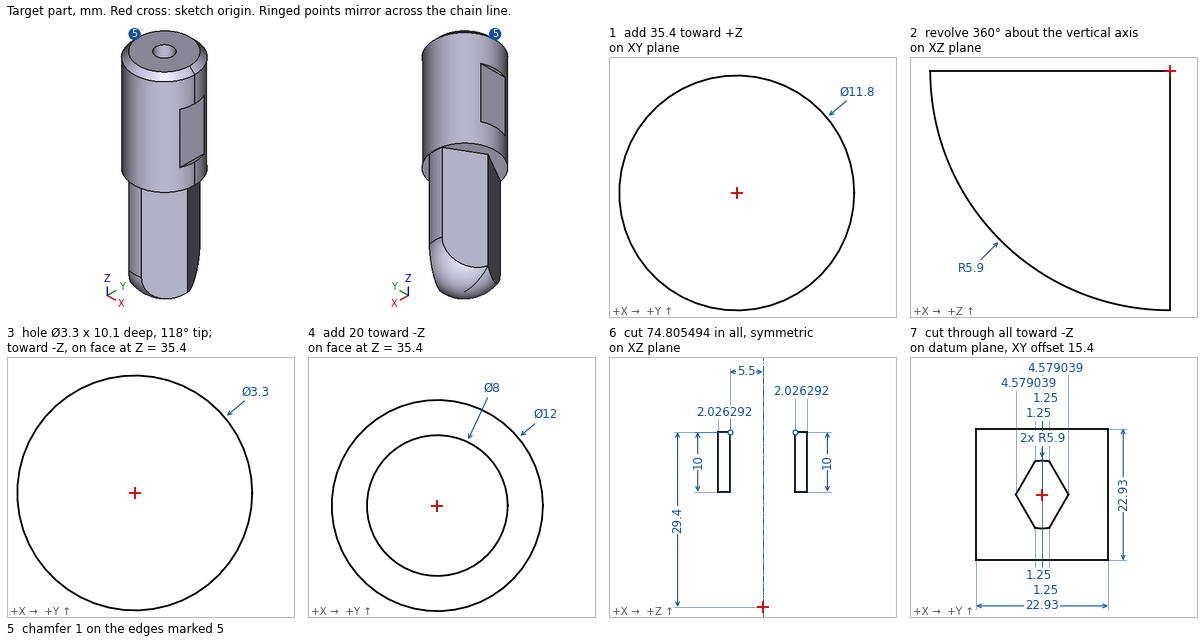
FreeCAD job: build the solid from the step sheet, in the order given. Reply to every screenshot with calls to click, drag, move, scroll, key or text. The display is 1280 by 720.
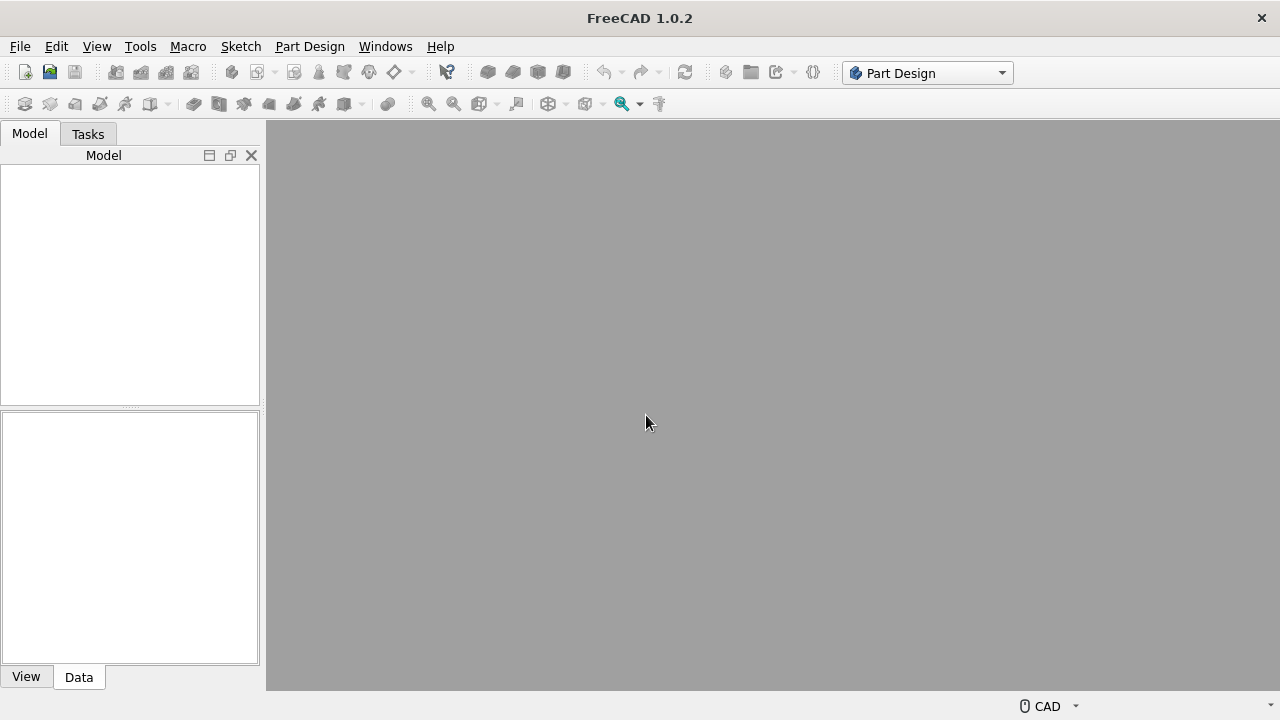
click(25, 72)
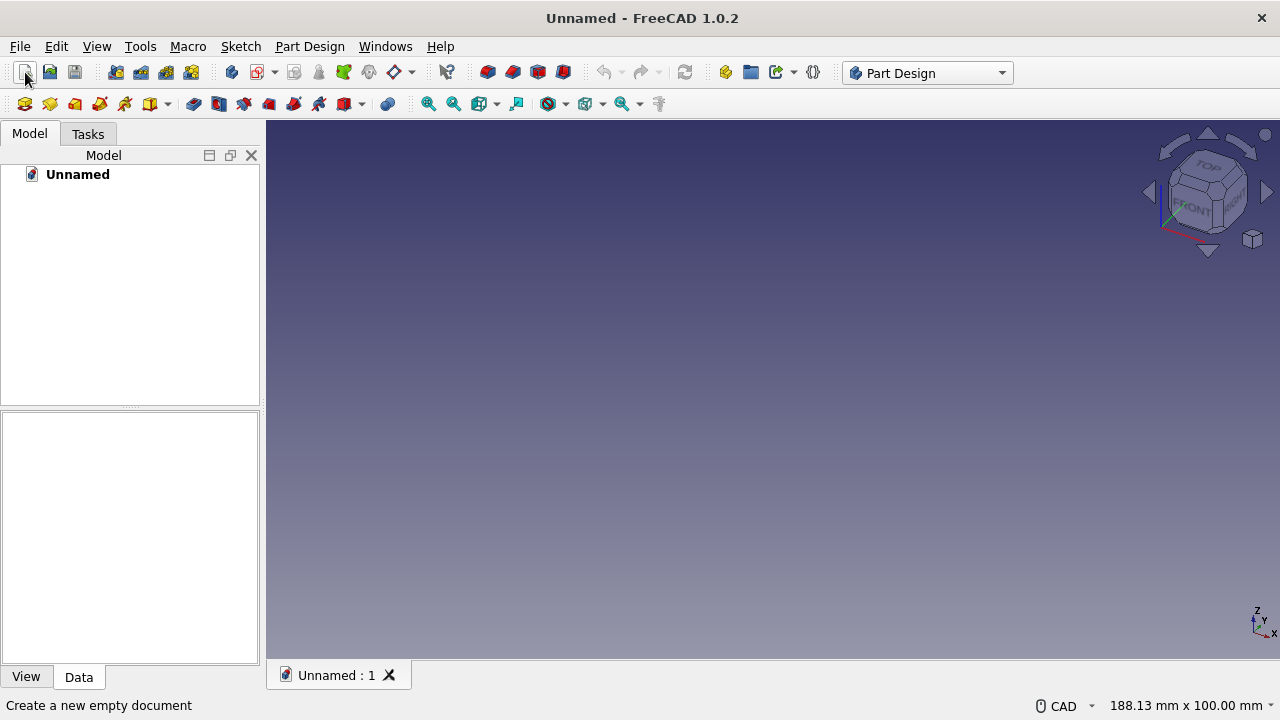
click(256, 72)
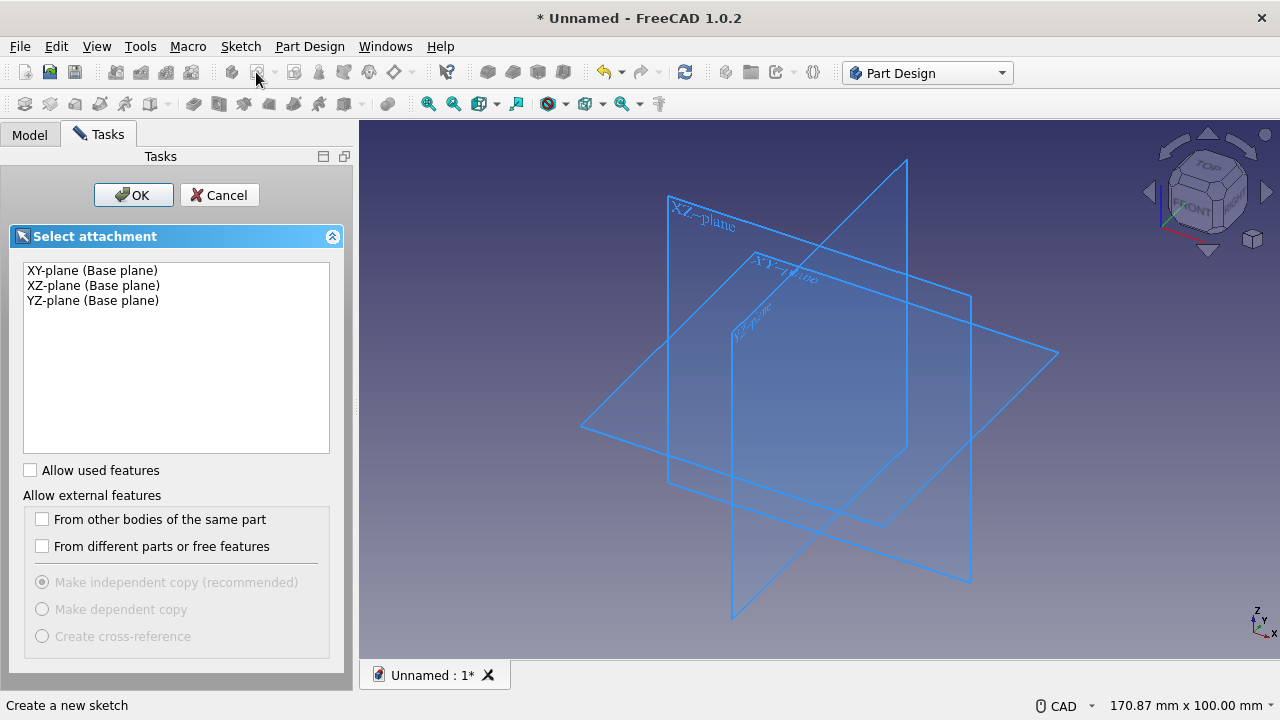
click(84, 270)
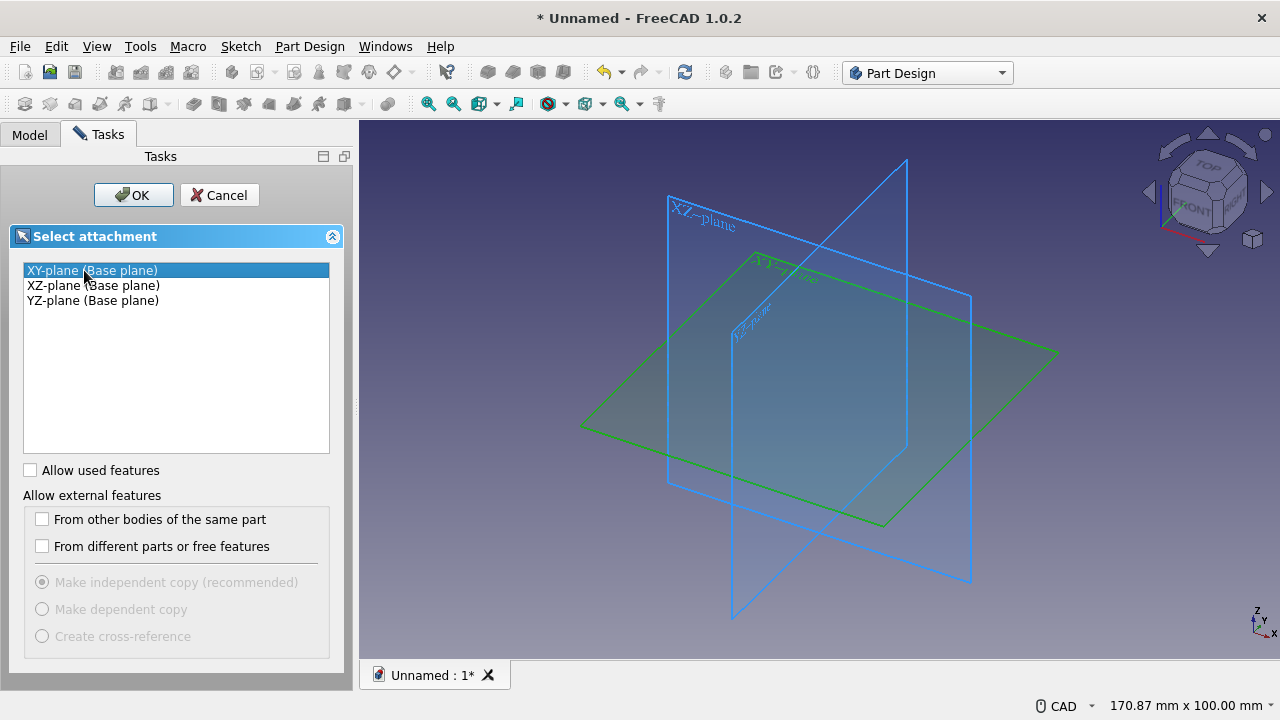
click(134, 195)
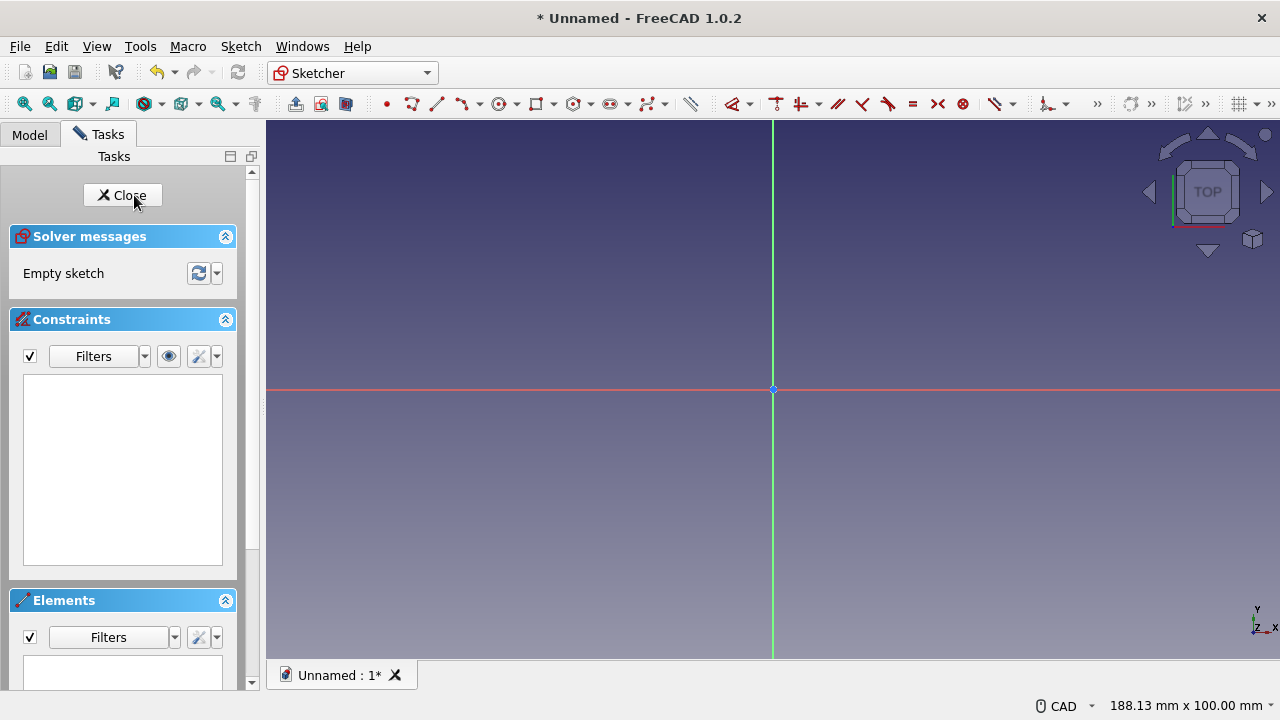
scroll(790, 390, up, 8)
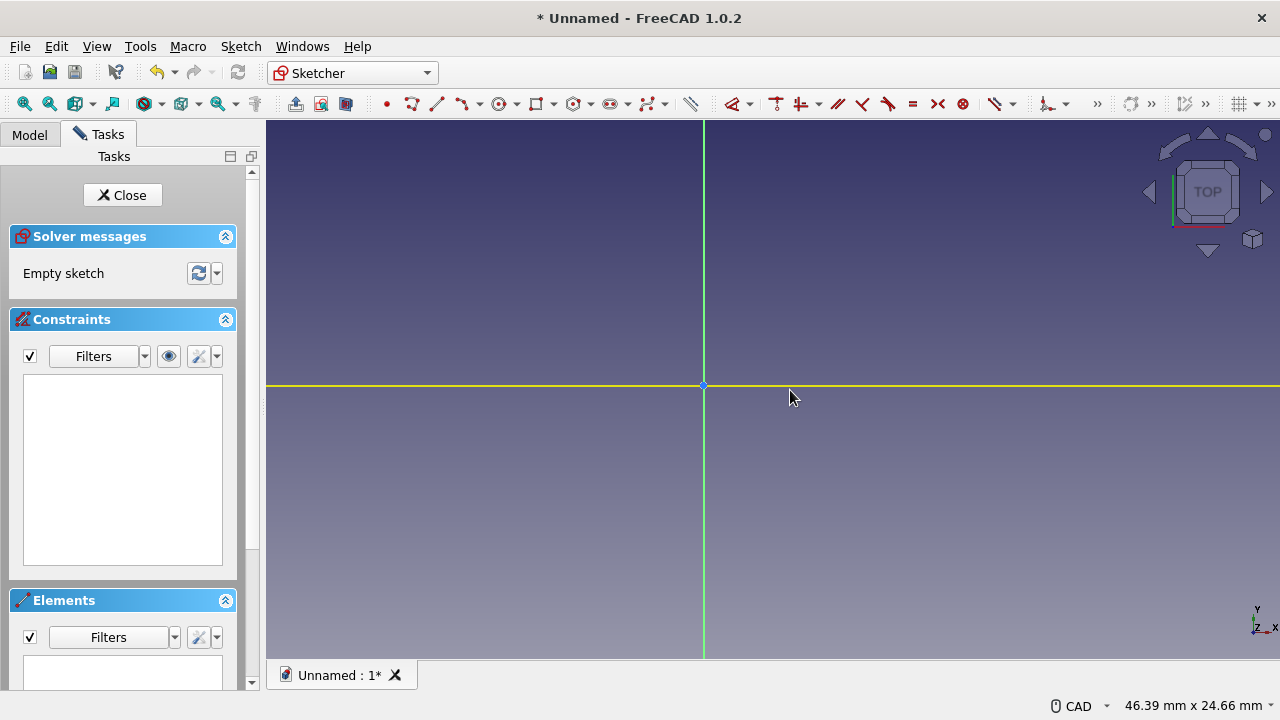
key(g)
key(c)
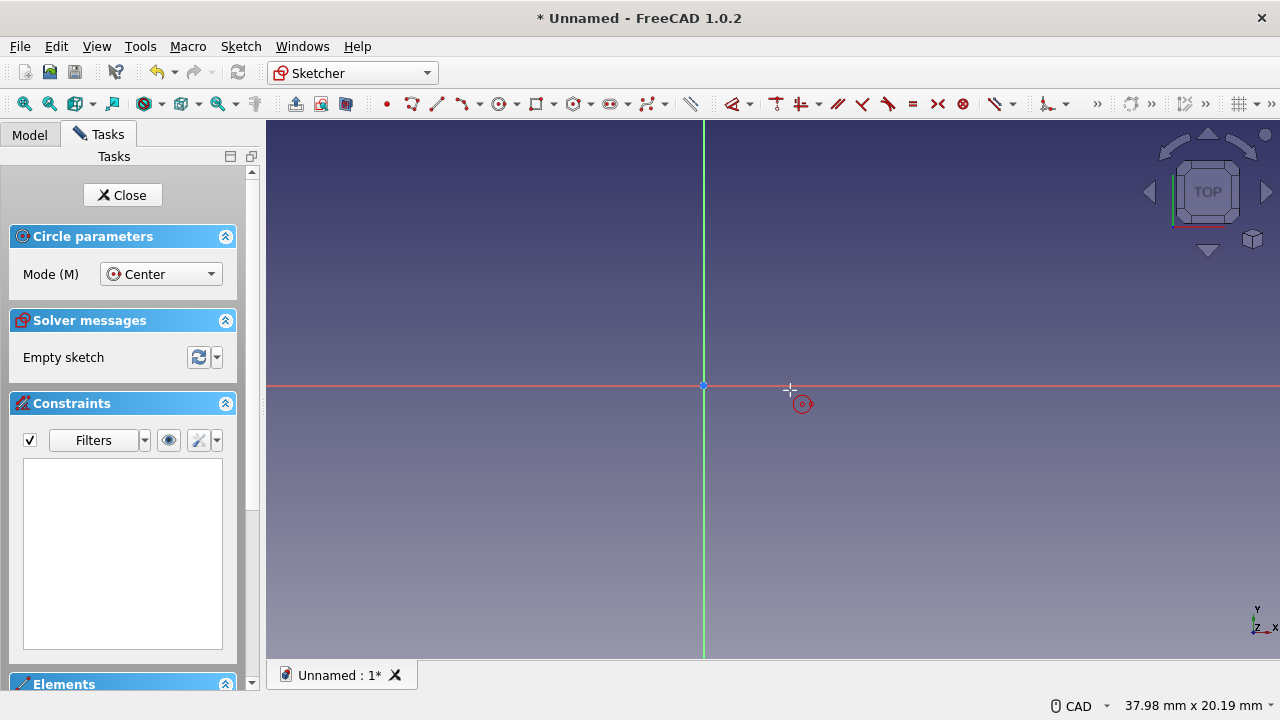
click(704, 386)
move(815, 274)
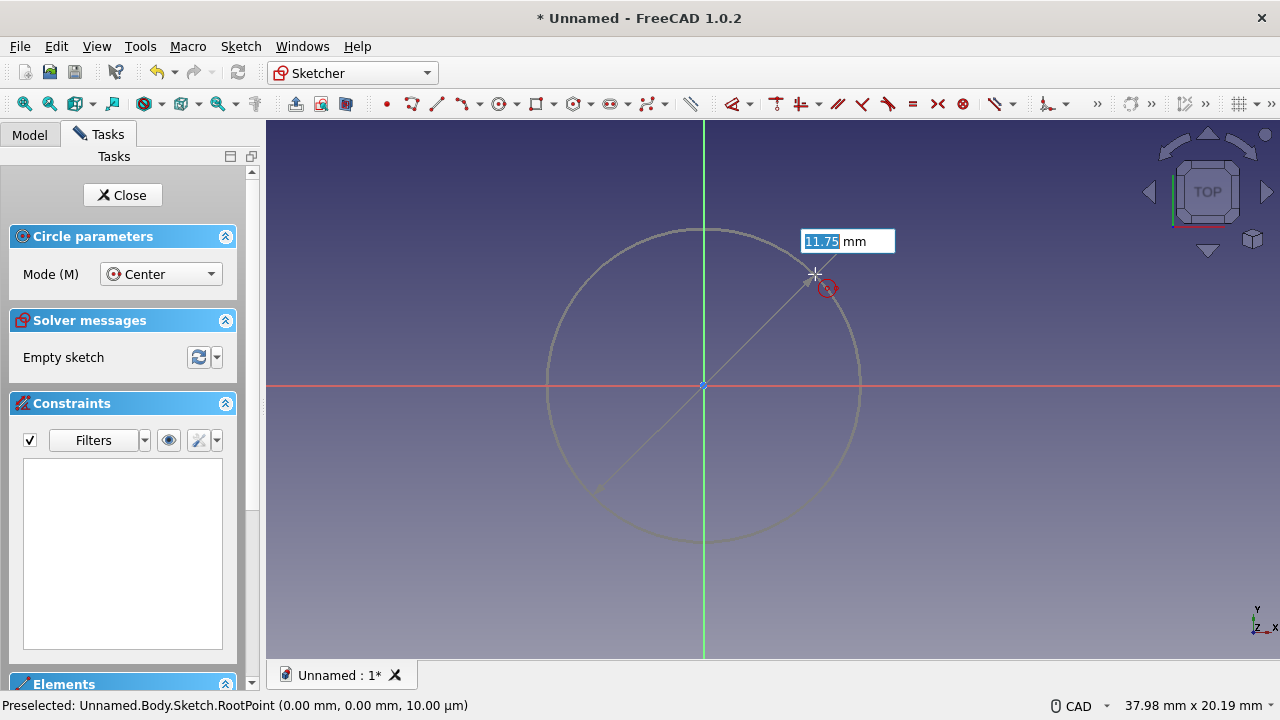
text(11.8)
key(Return)
key(Escape)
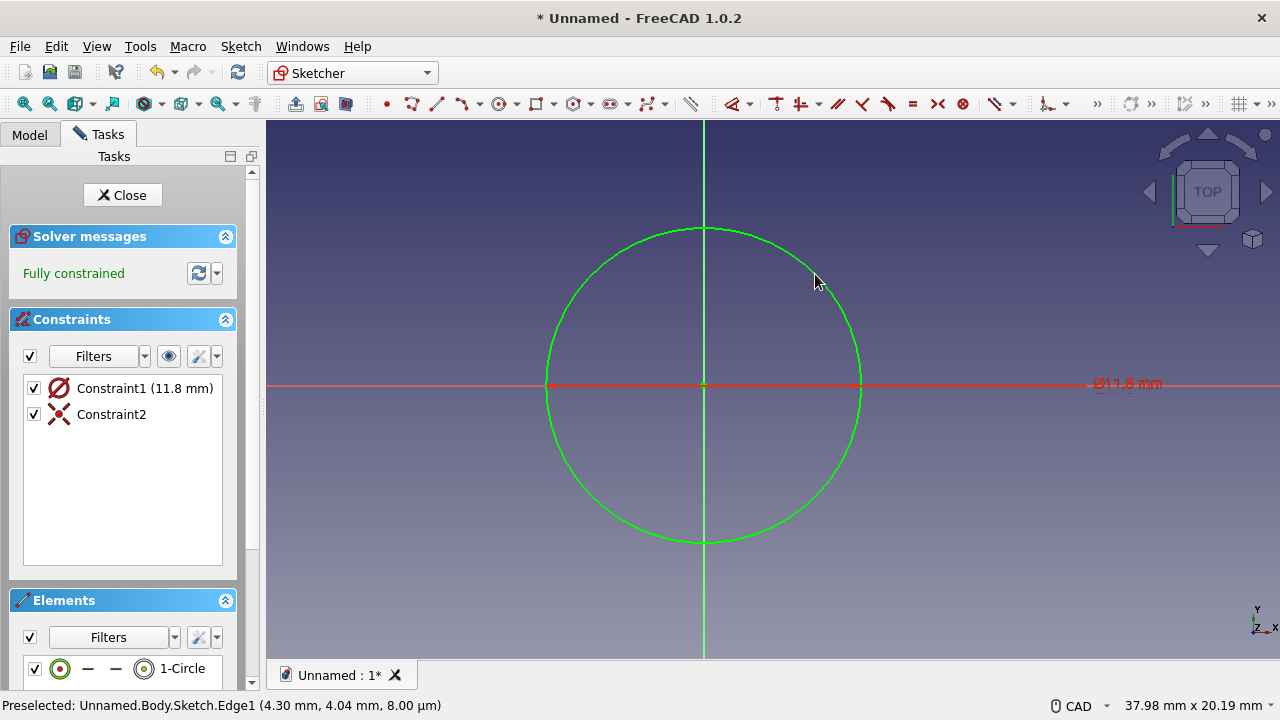
click(123, 195)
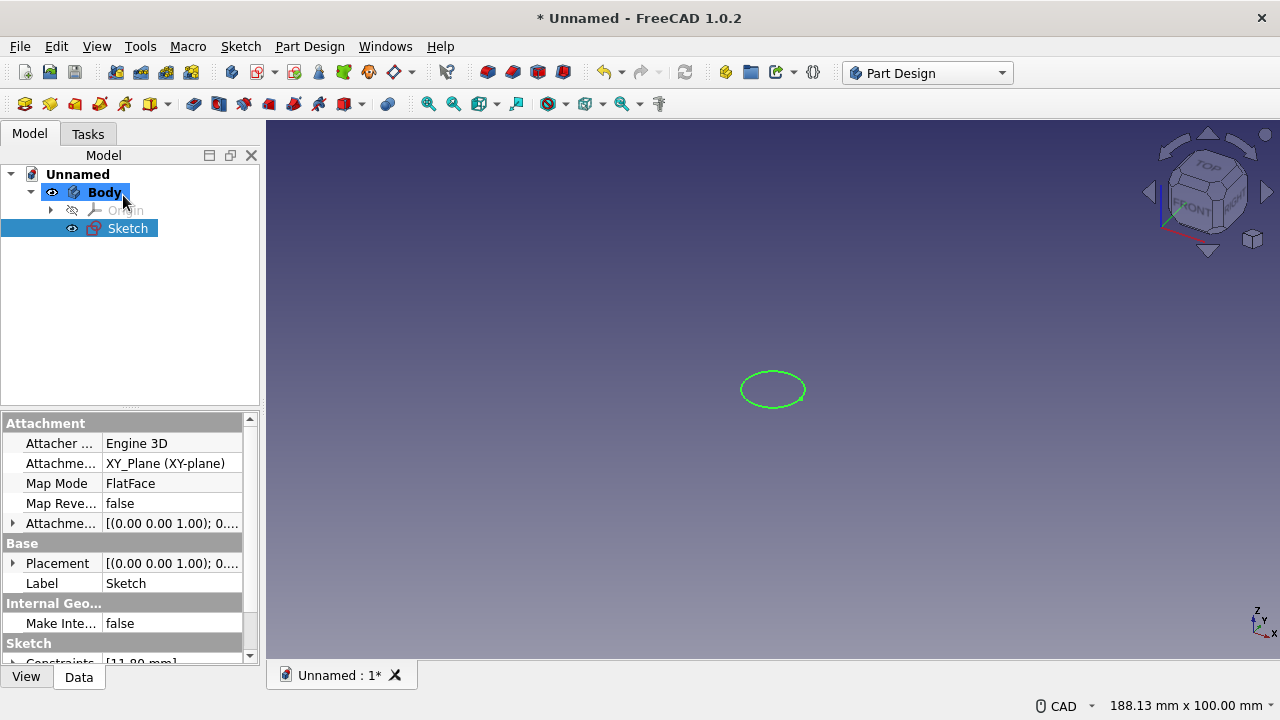
click(25, 104)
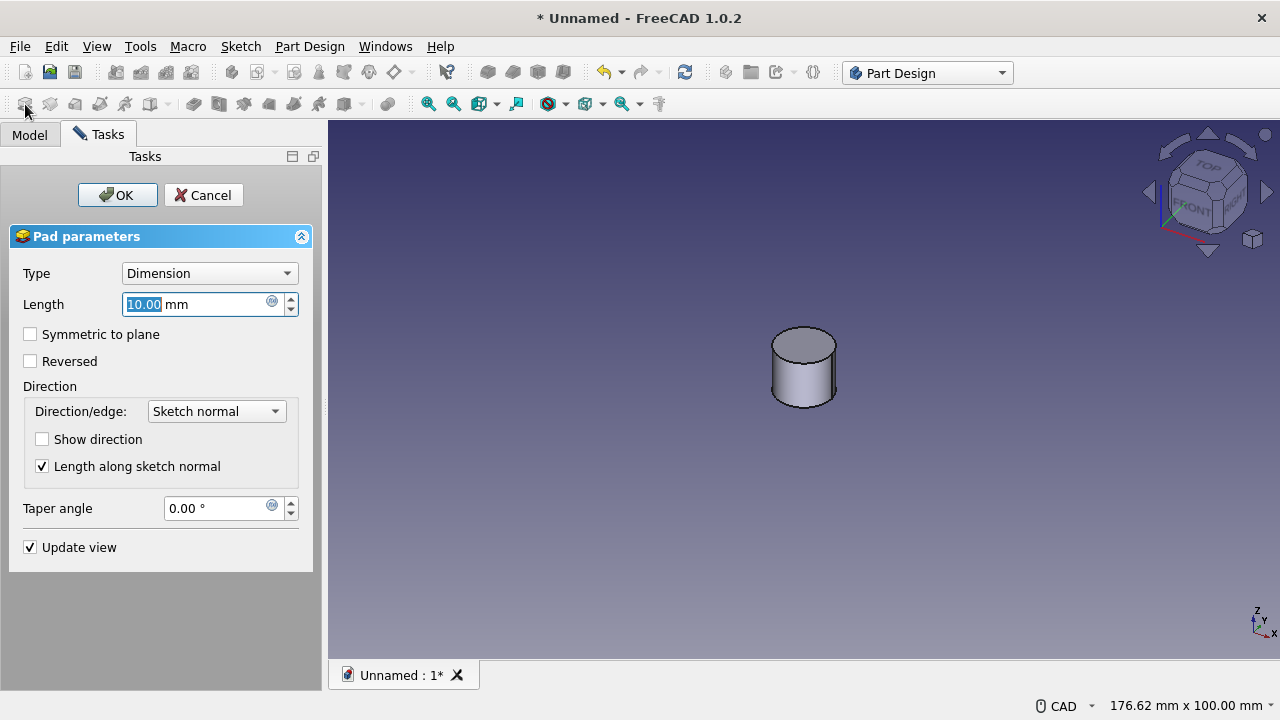
text(35.4)
key(Tab)